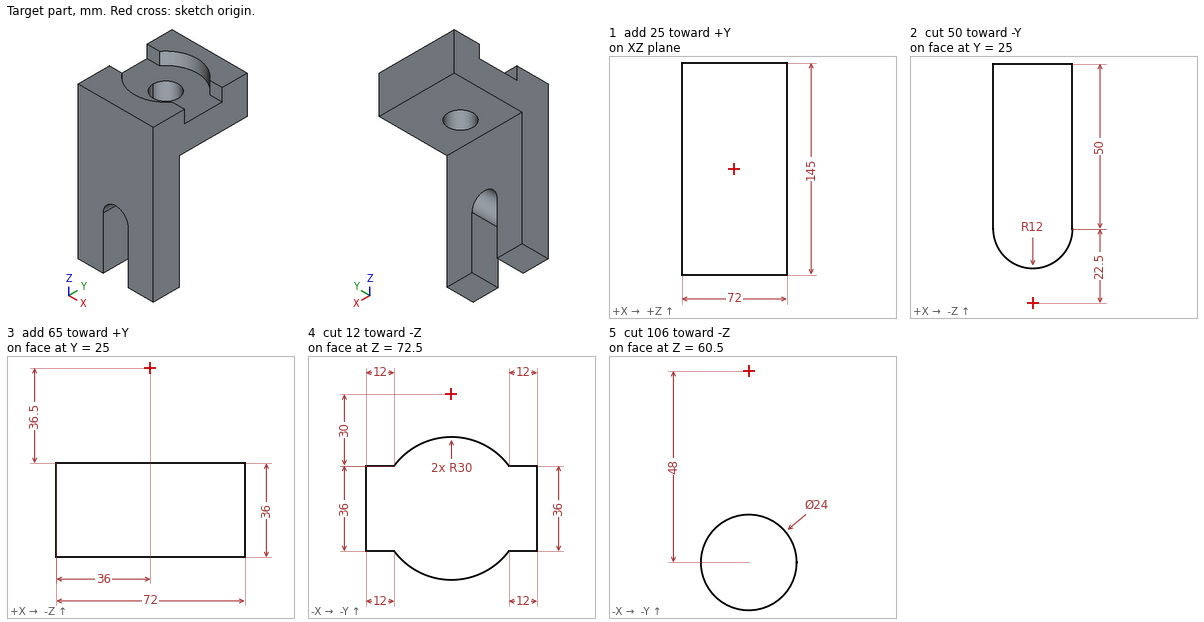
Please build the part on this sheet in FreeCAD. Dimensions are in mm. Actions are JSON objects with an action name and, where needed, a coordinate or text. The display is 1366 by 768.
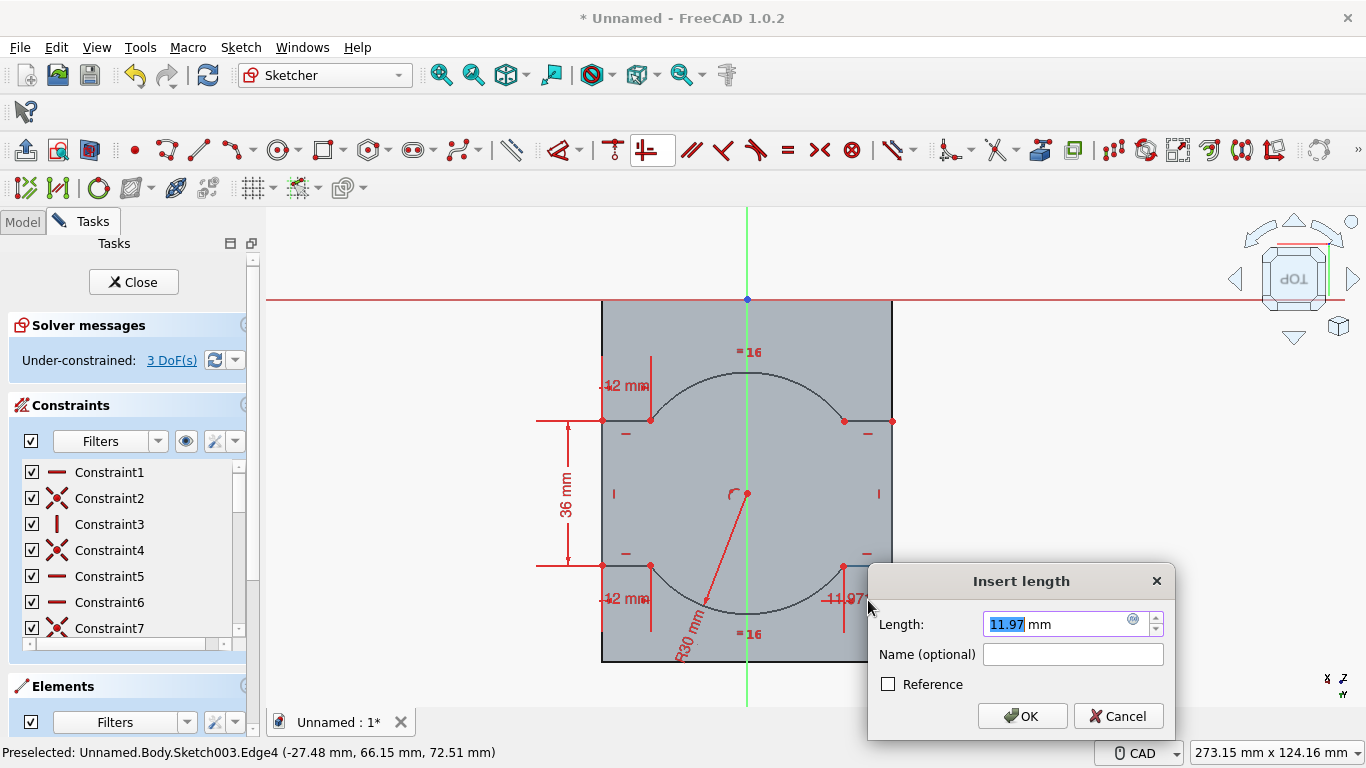
{"action": "type", "text": "12"}
{"action": "key", "text": "Return"}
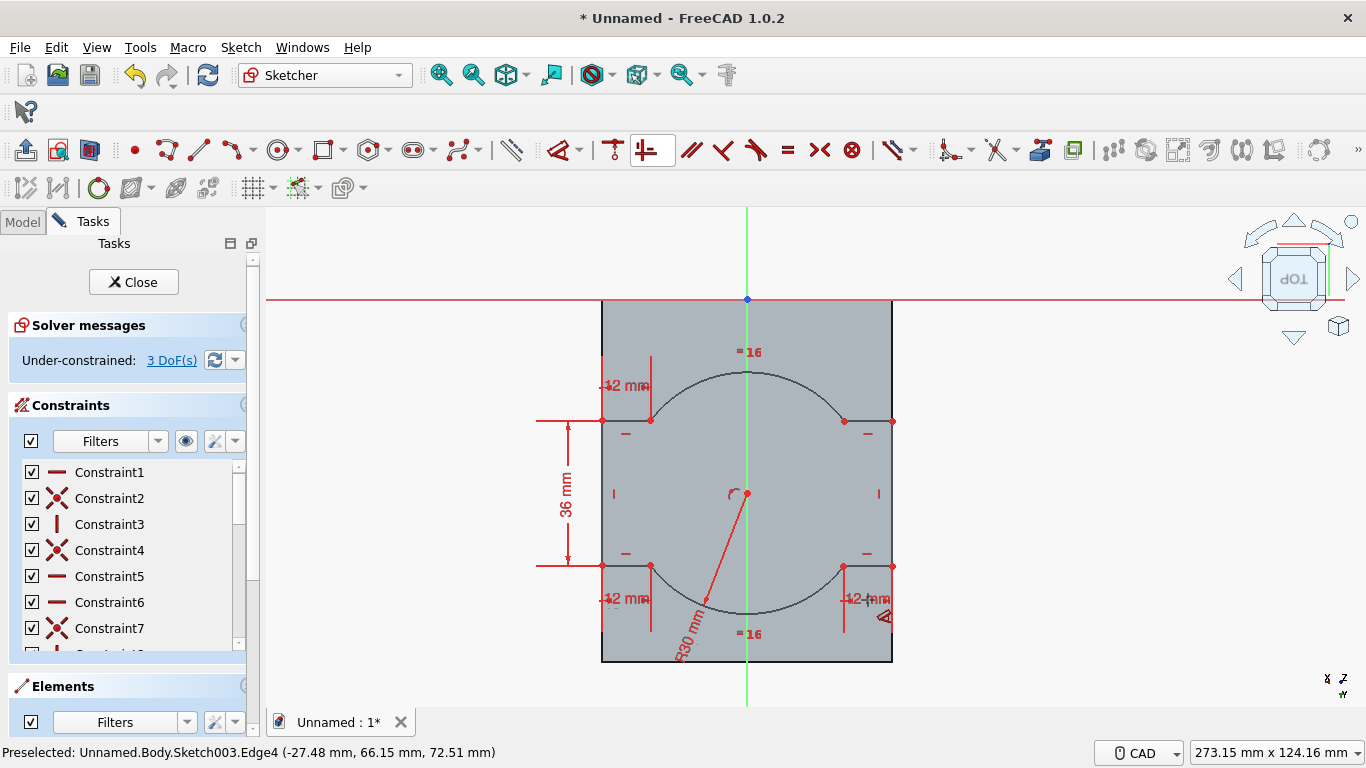
{"action": "left_click", "coordinate": [892, 523]}
{"action": "left_click", "coordinate": [926, 494]}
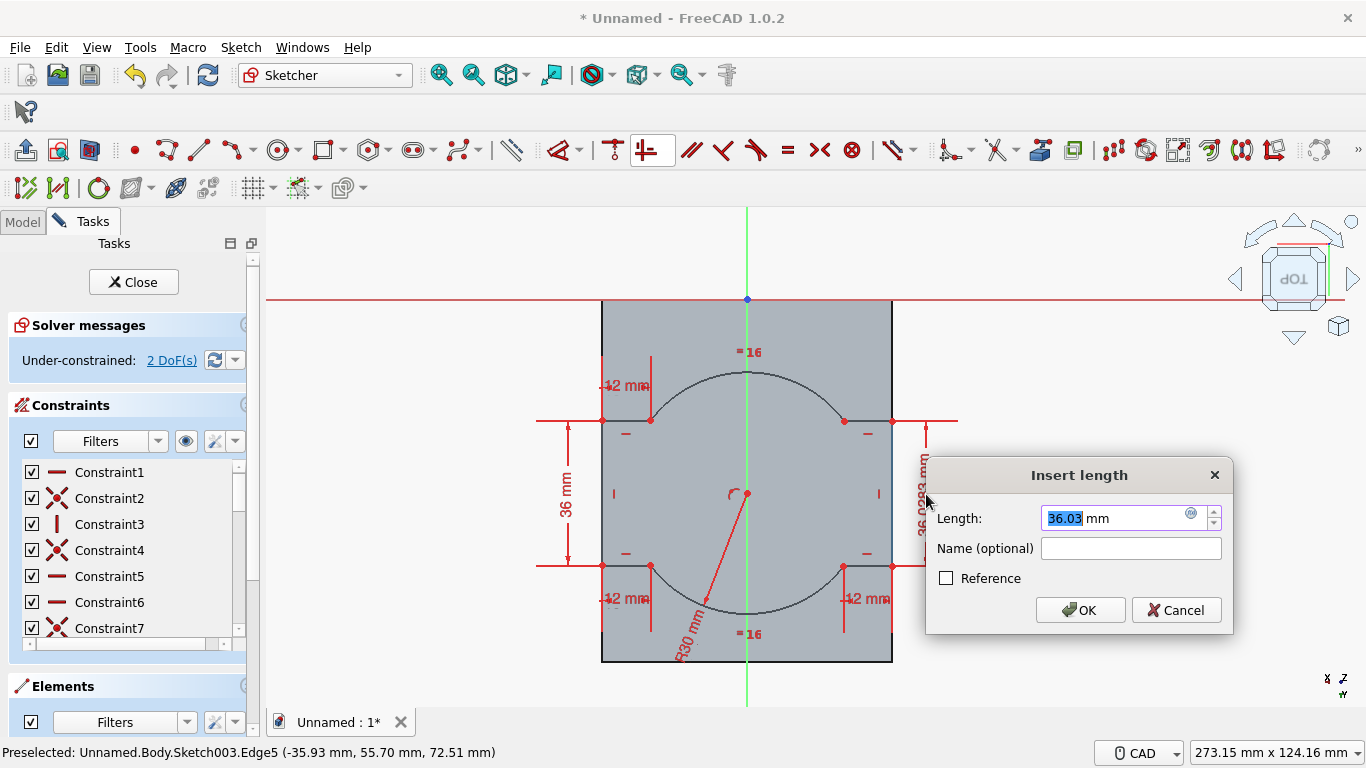
{"action": "type", "text": "36"}
{"action": "key", "text": "Return"}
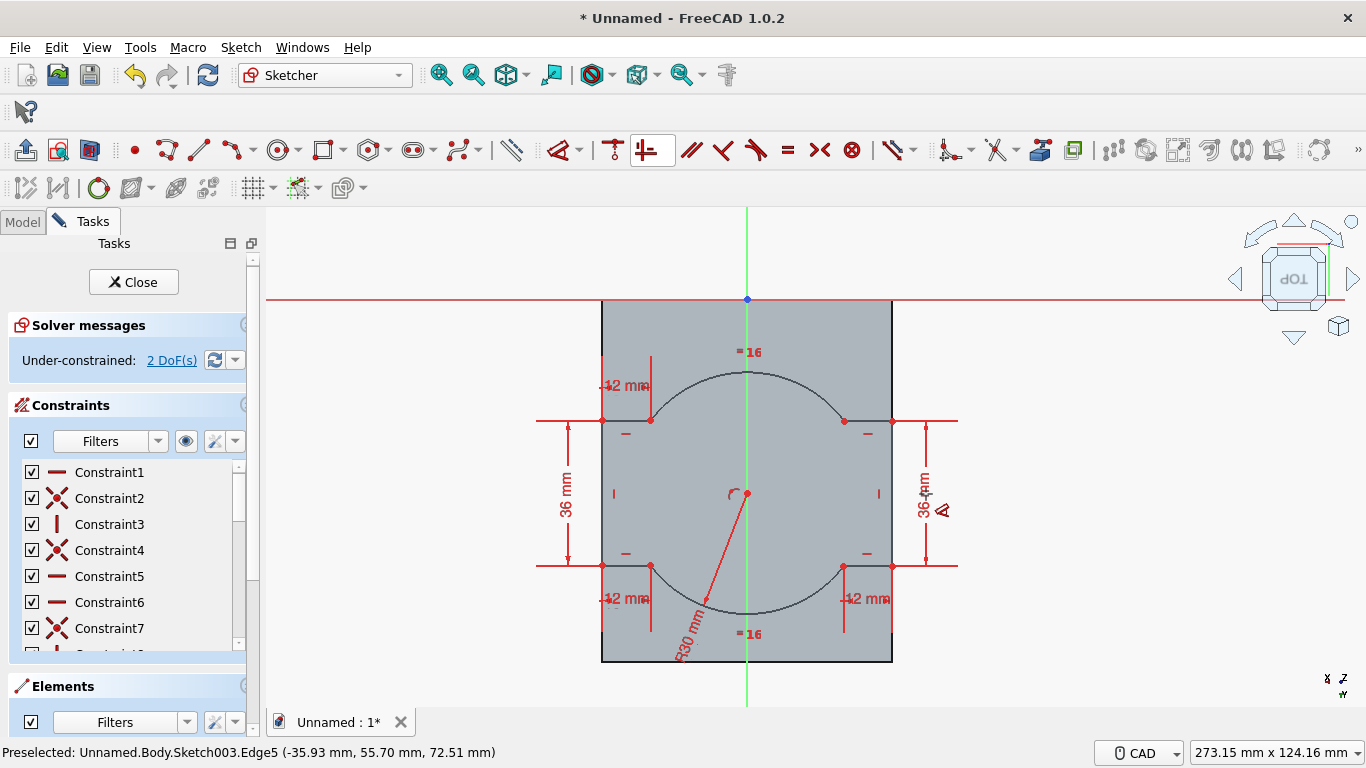
{"action": "left_click", "coordinate": [878, 421]}
{"action": "left_click", "coordinate": [868, 387]}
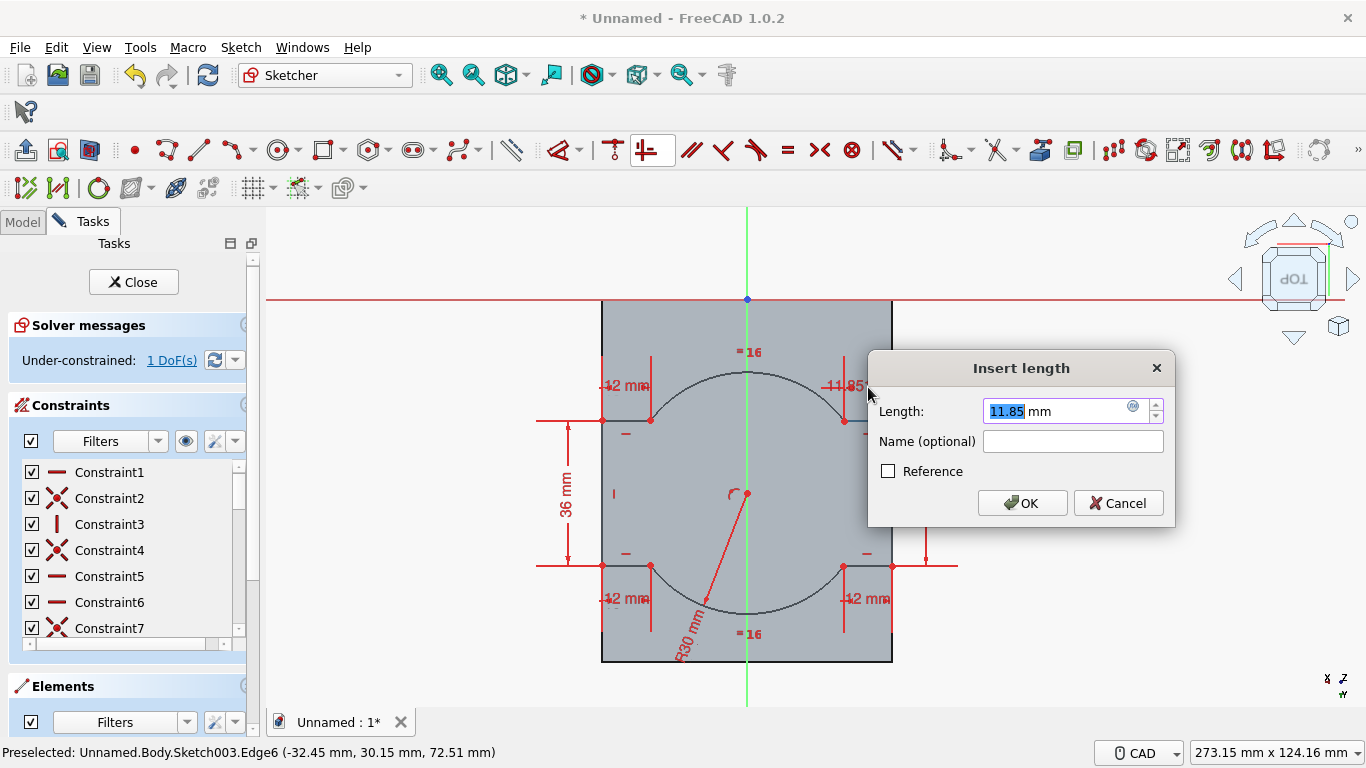
{"action": "type", "text": "12"}
{"action": "key", "text": "Return"}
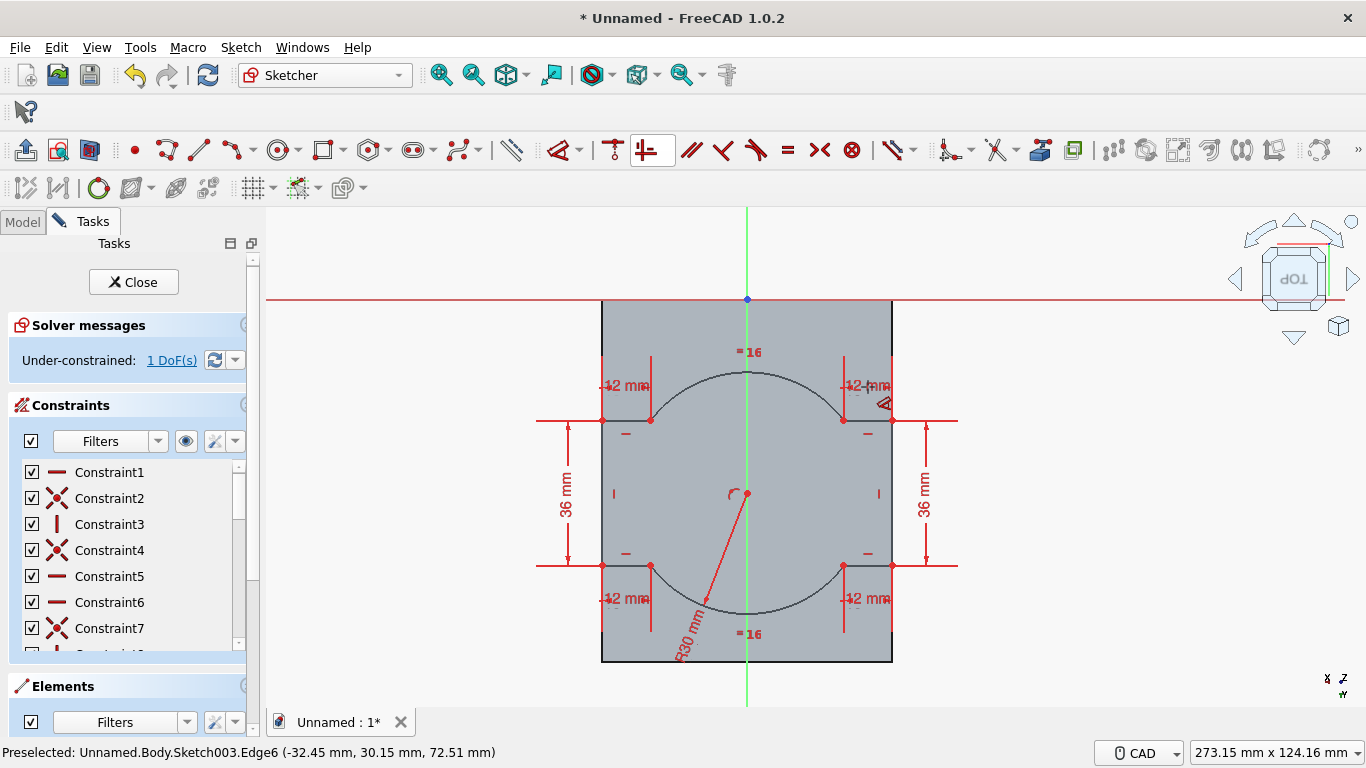
{"action": "left_click", "coordinate": [651, 421]}
{"action": "left_click", "coordinate": [617, 360]}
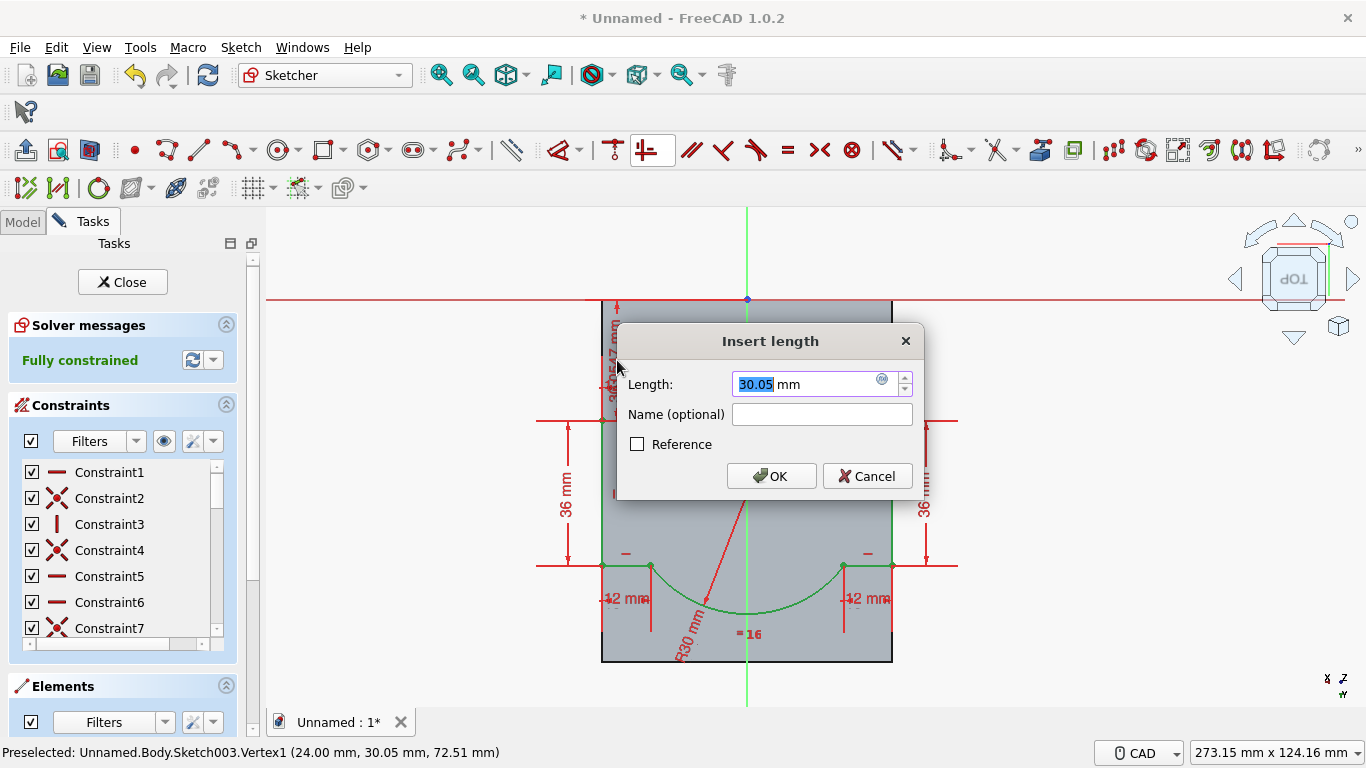
{"action": "type", "text": "30"}
{"action": "key", "text": "Return"}
{"action": "key", "text": "Escape"}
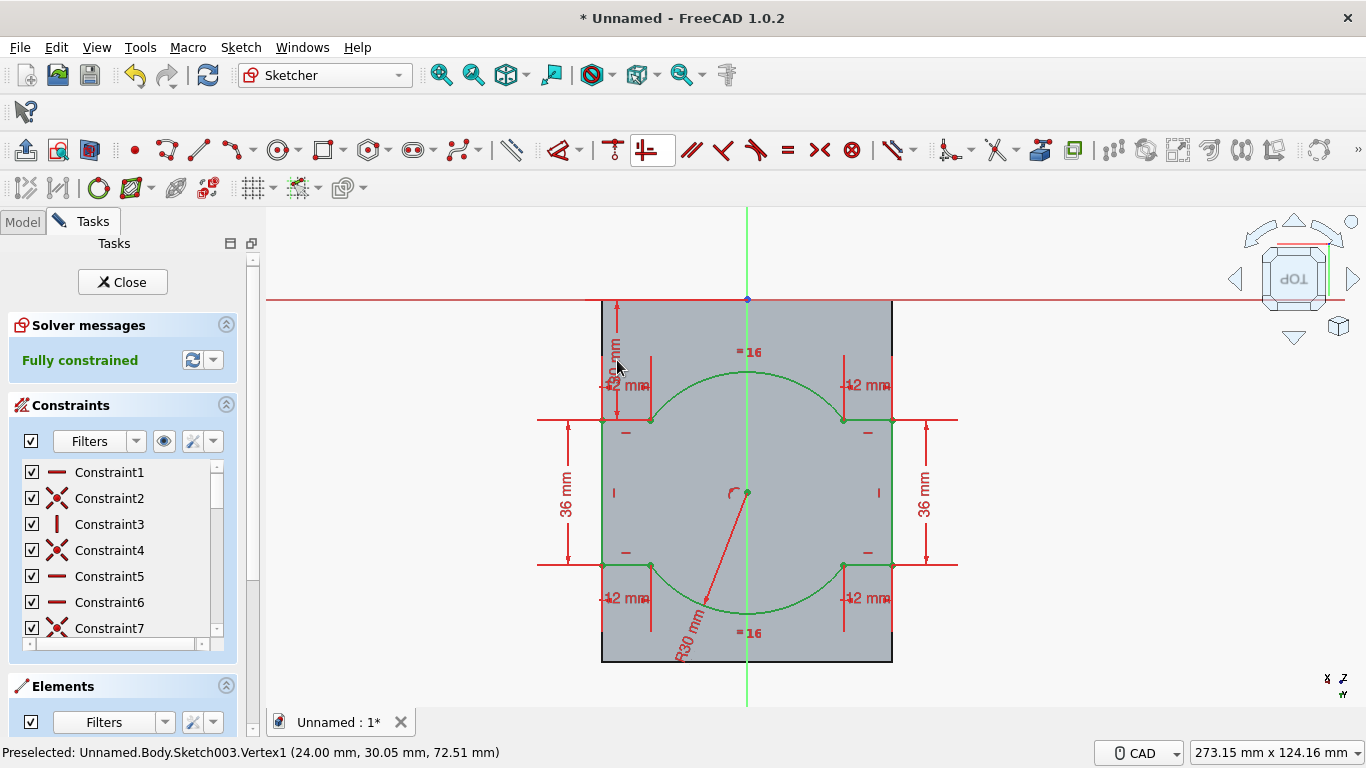
{"action": "left_click", "coordinate": [123, 282]}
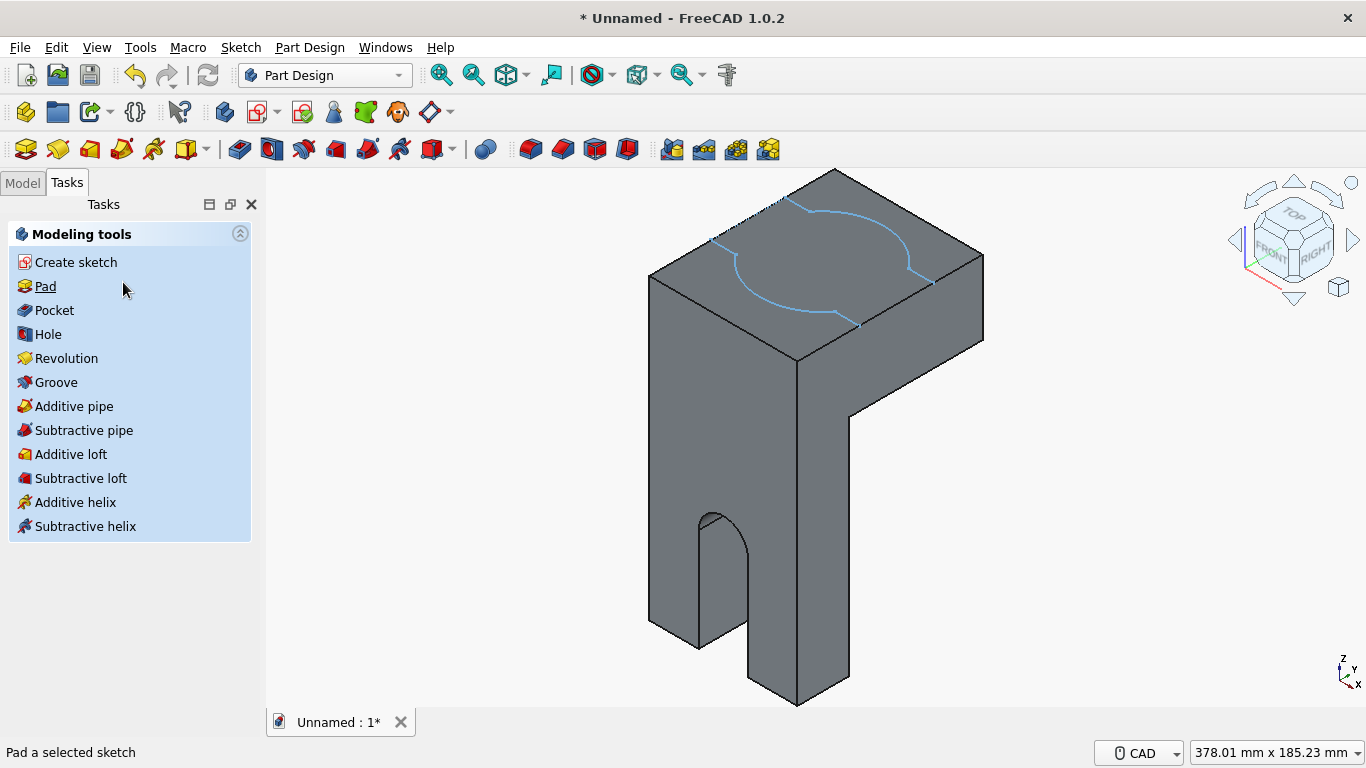
{"action": "left_click", "coordinate": [240, 150]}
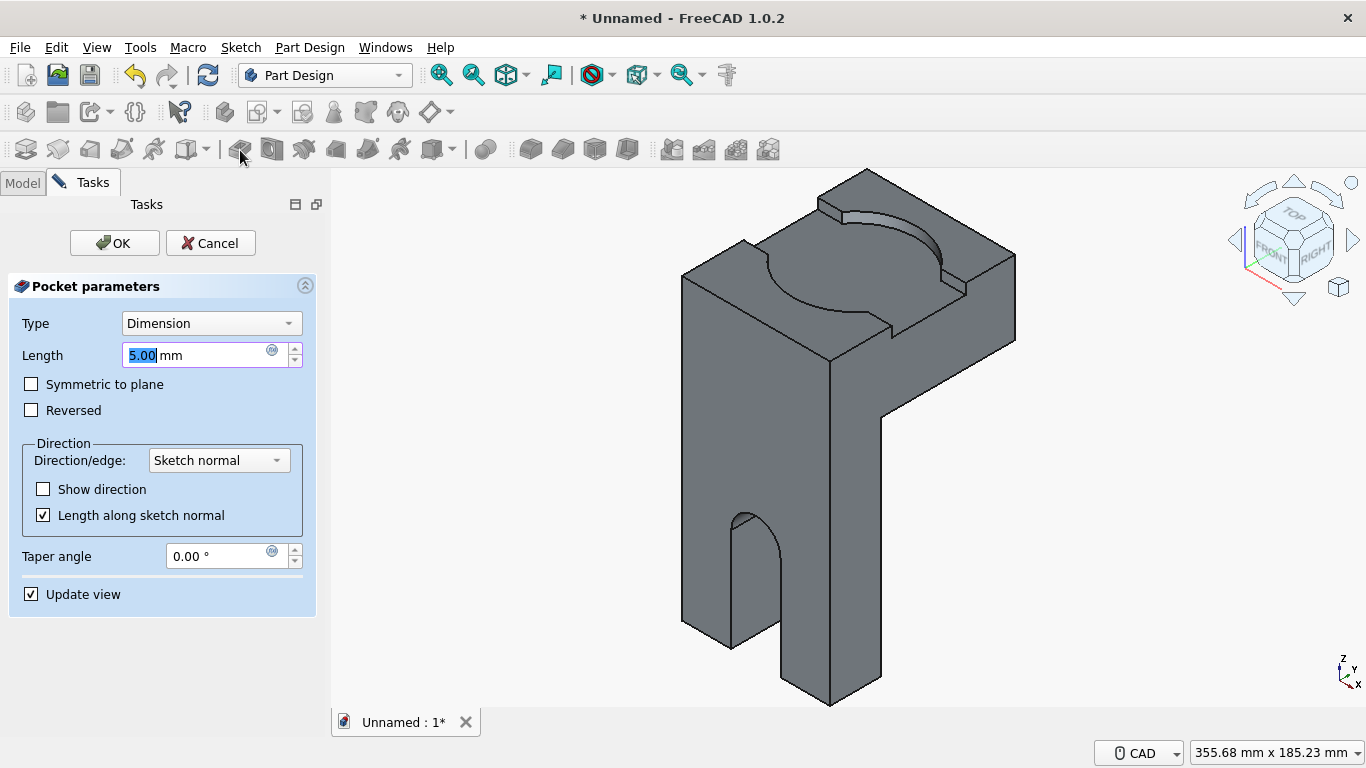
{"action": "type", "text": "12"}
{"action": "key", "text": "Tab"}